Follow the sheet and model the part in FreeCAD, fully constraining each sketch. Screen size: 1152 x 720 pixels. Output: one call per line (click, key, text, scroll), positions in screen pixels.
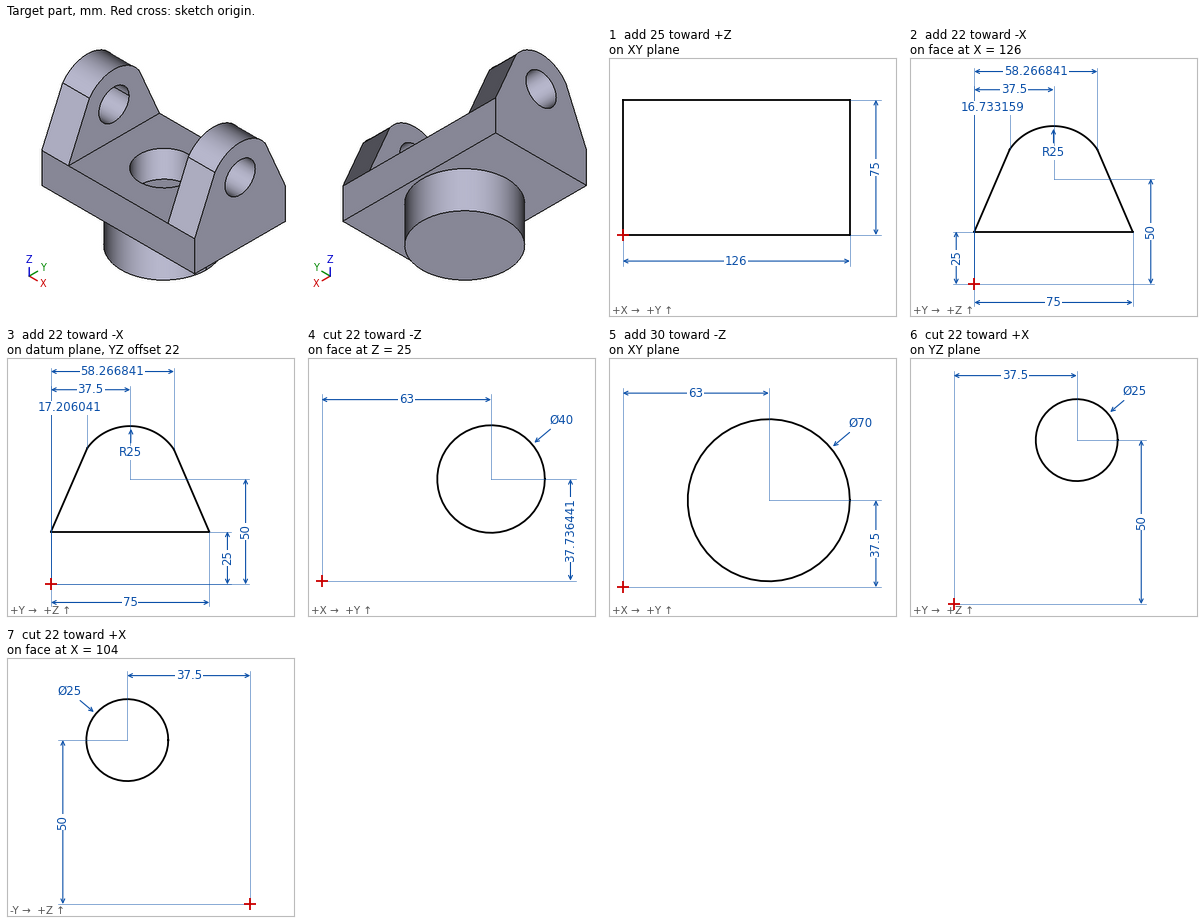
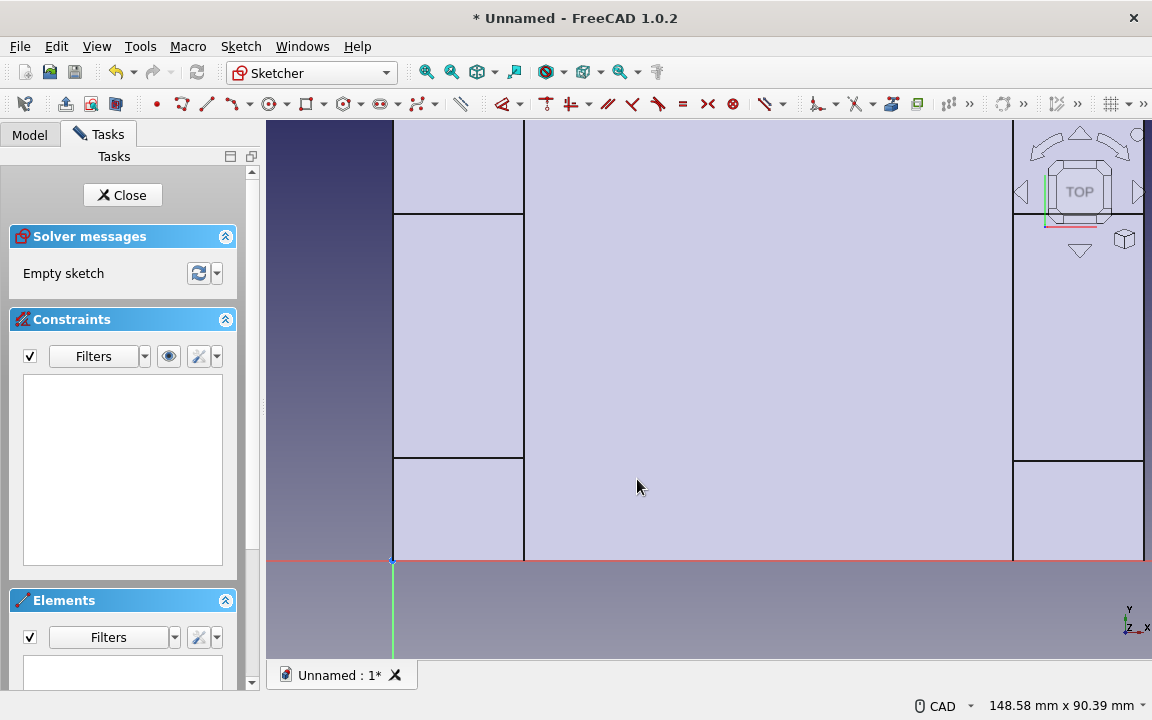
click(268, 104)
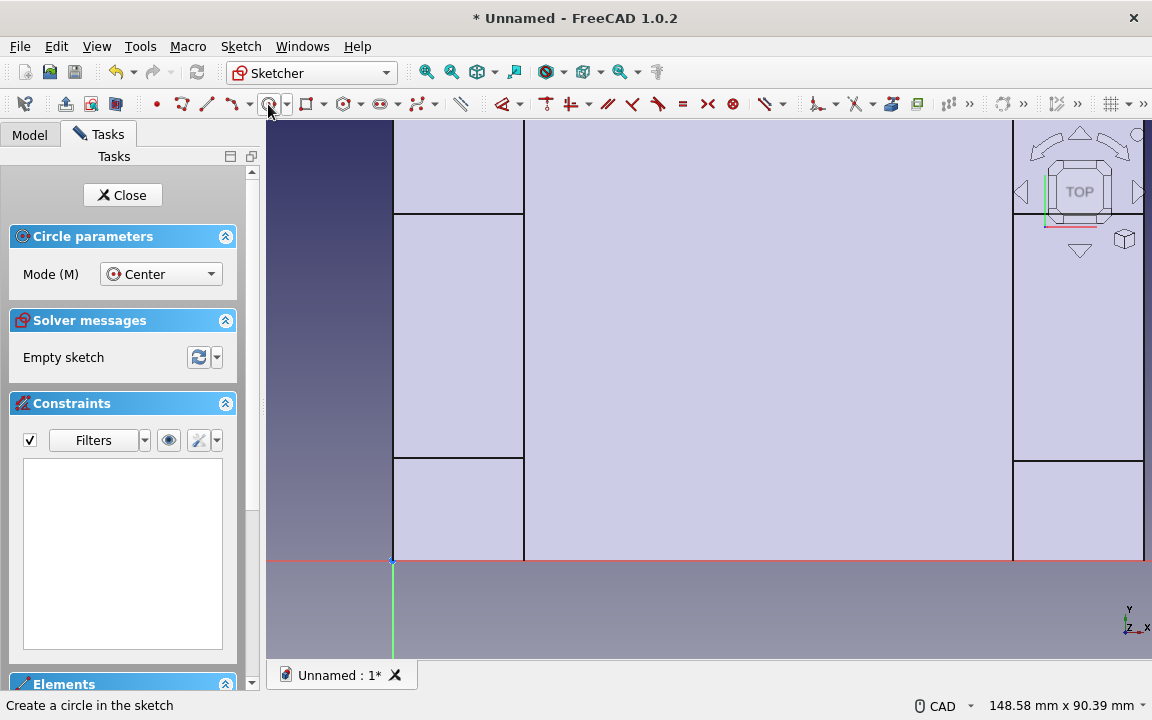
click(768, 336)
move(853, 252)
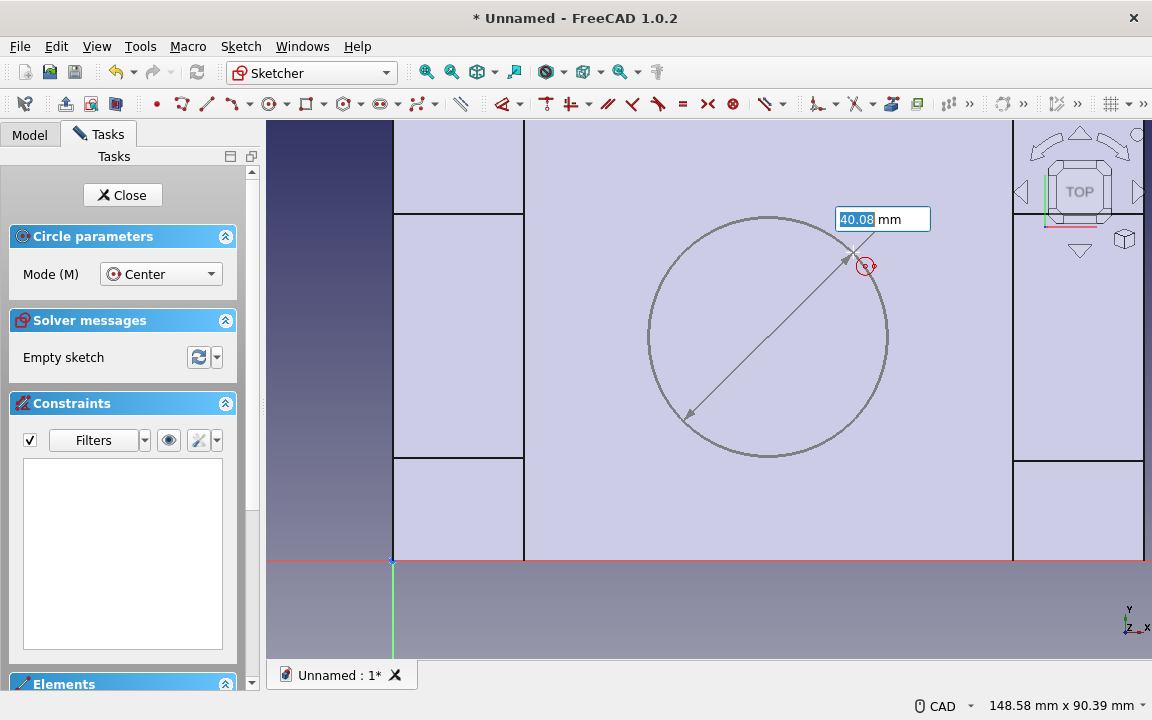
text(40)
key(Return)
key(Escape)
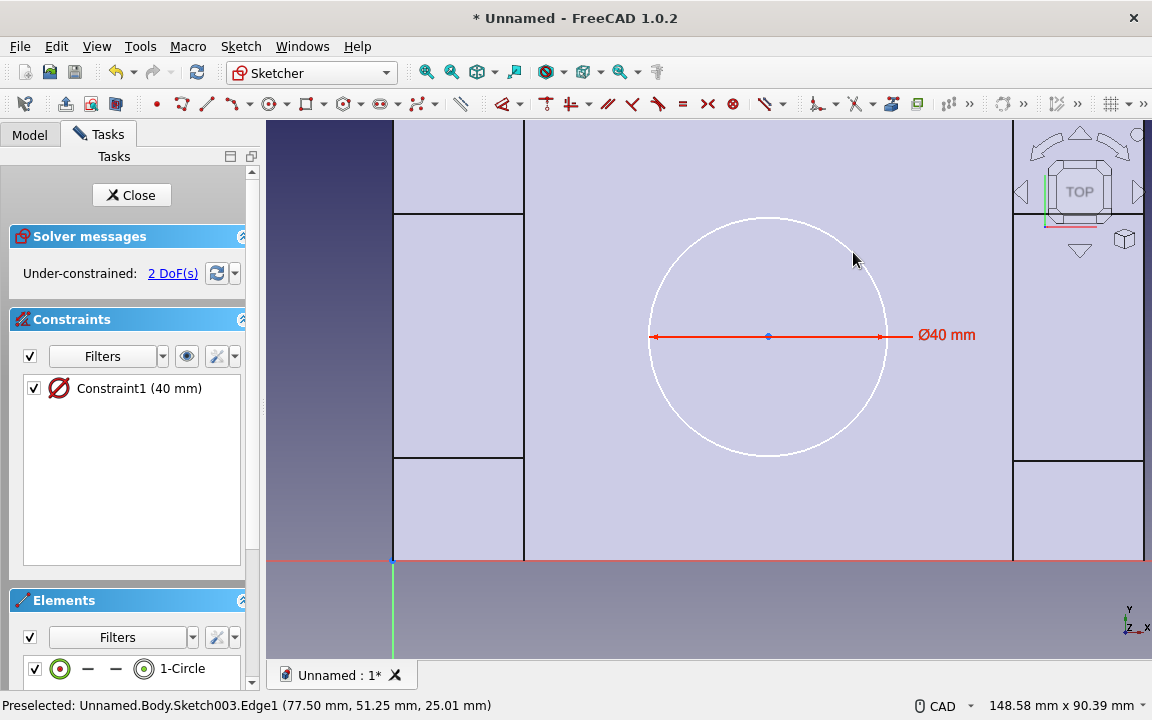
click(502, 104)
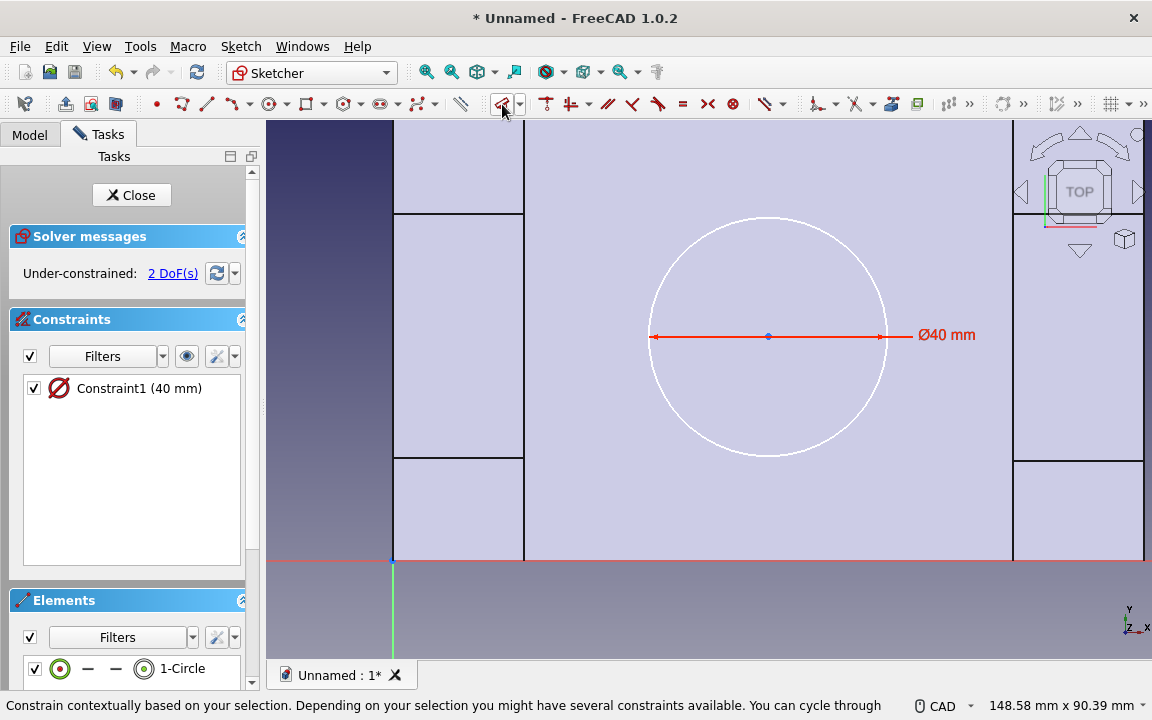
click(768, 337)
click(580, 595)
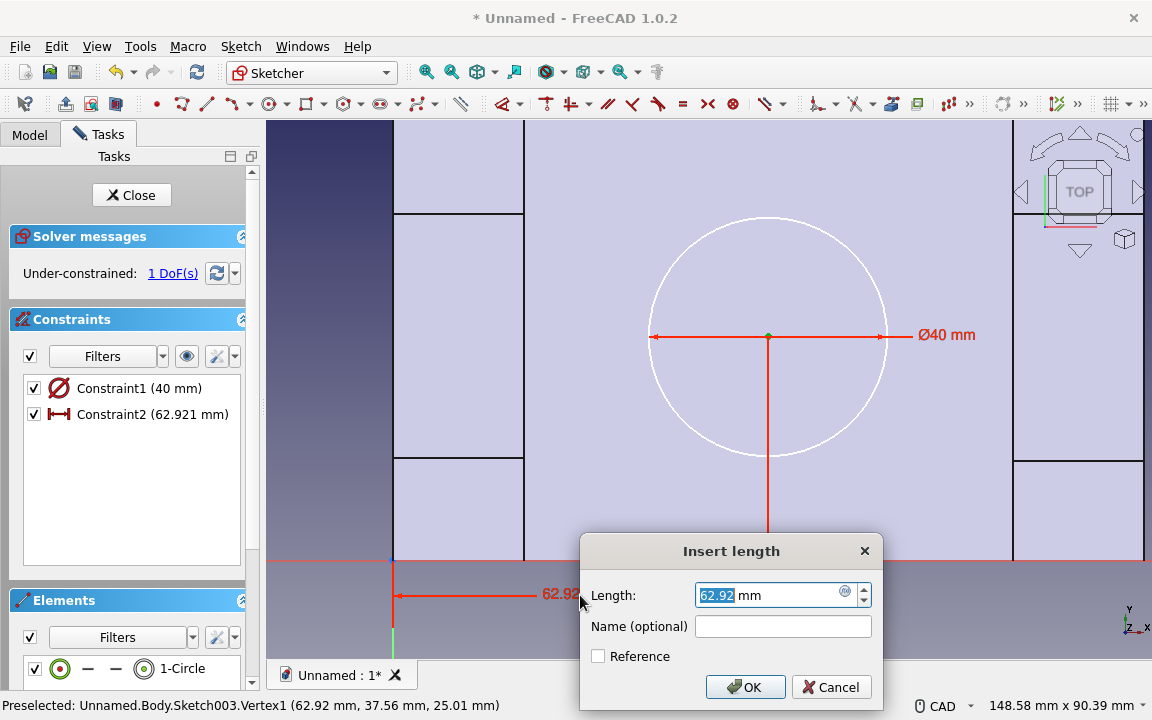
text(63)
key(Return)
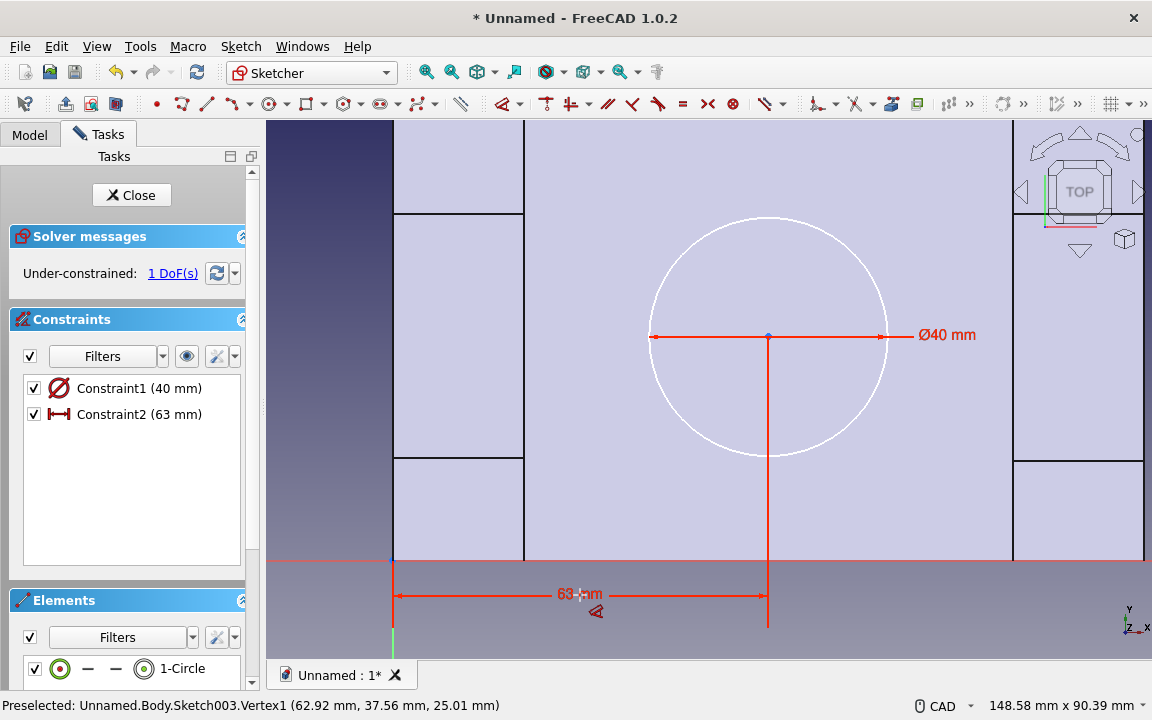
click(768, 337)
click(359, 449)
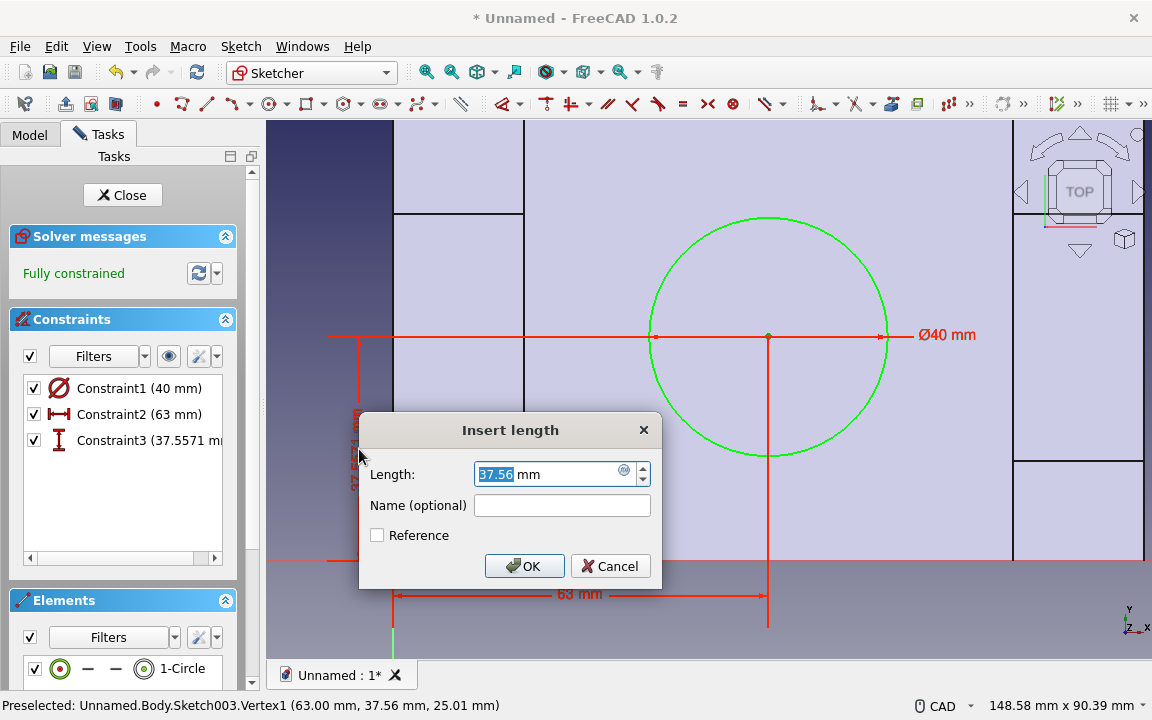
text(37.736441)
key(Return)
key(Escape)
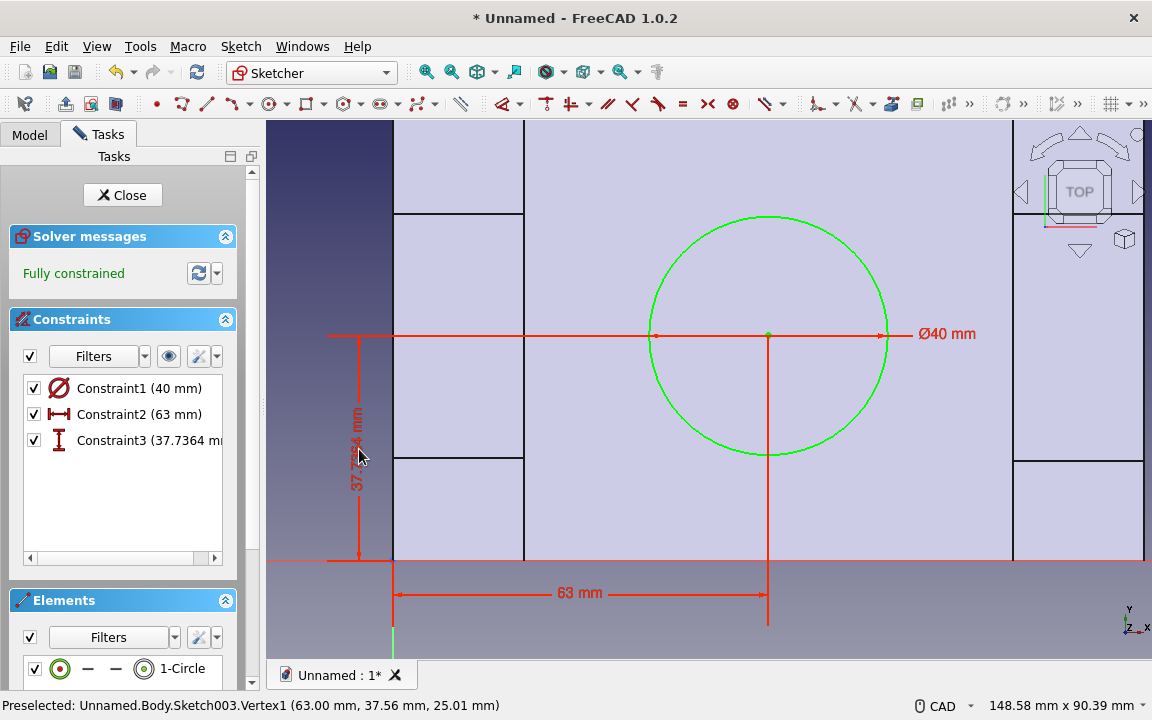
click(123, 195)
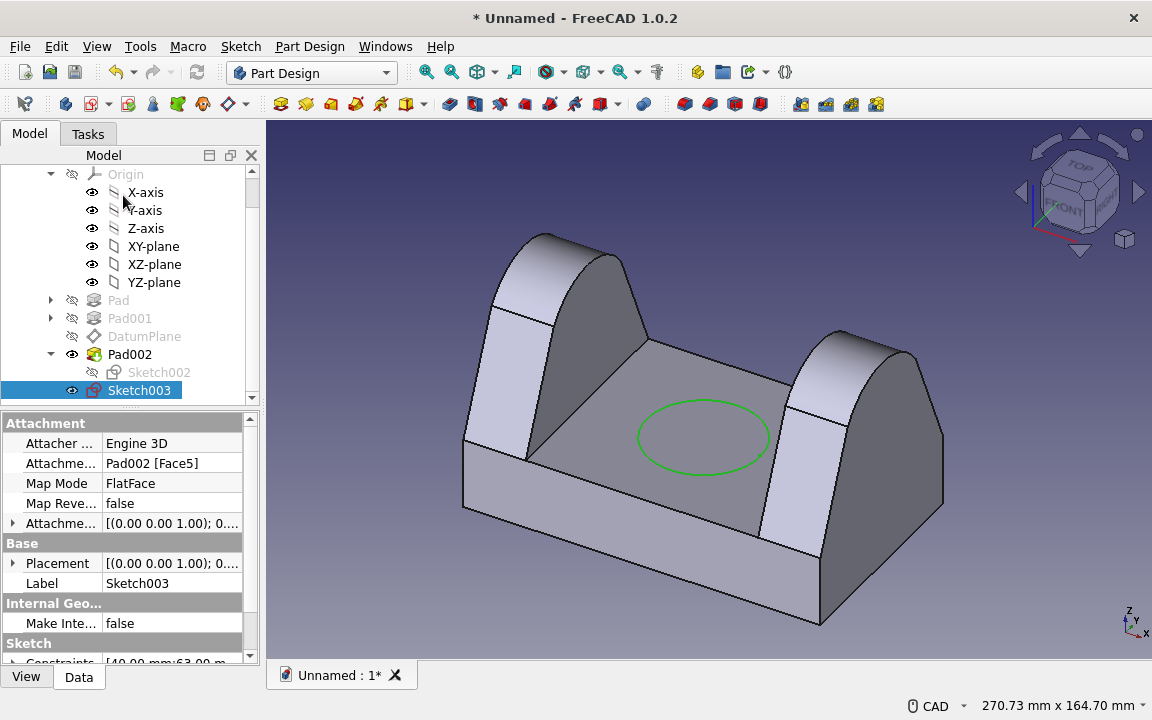
click(450, 104)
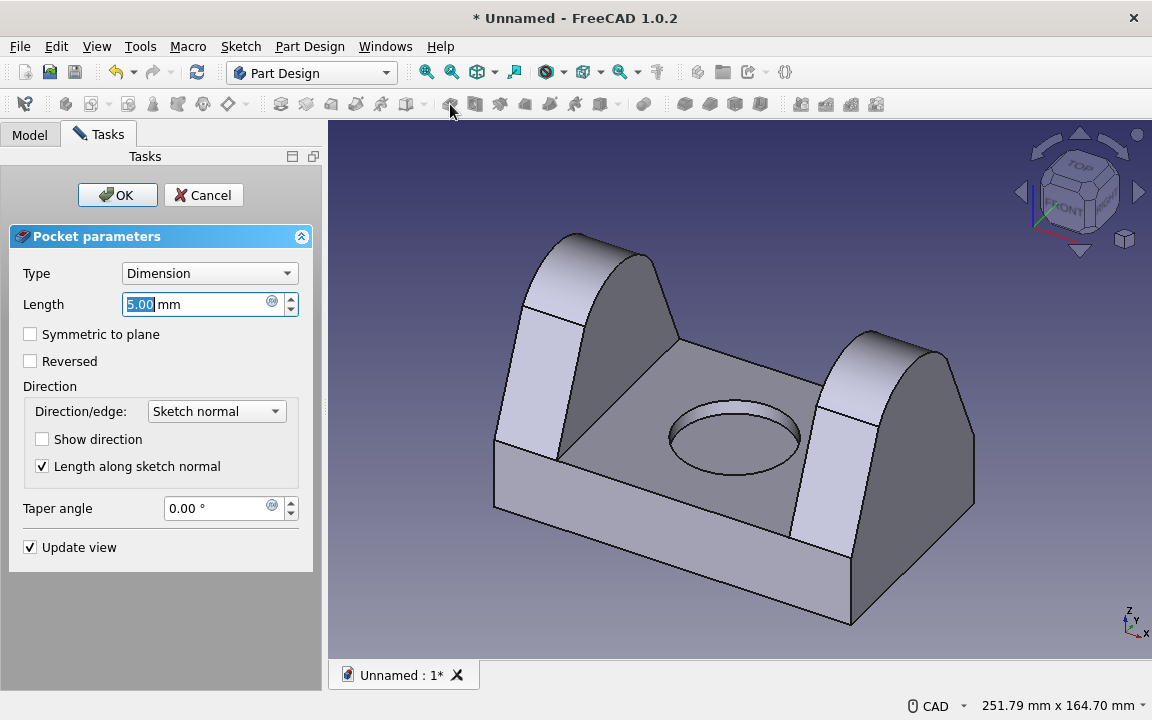
text(22)
key(Tab)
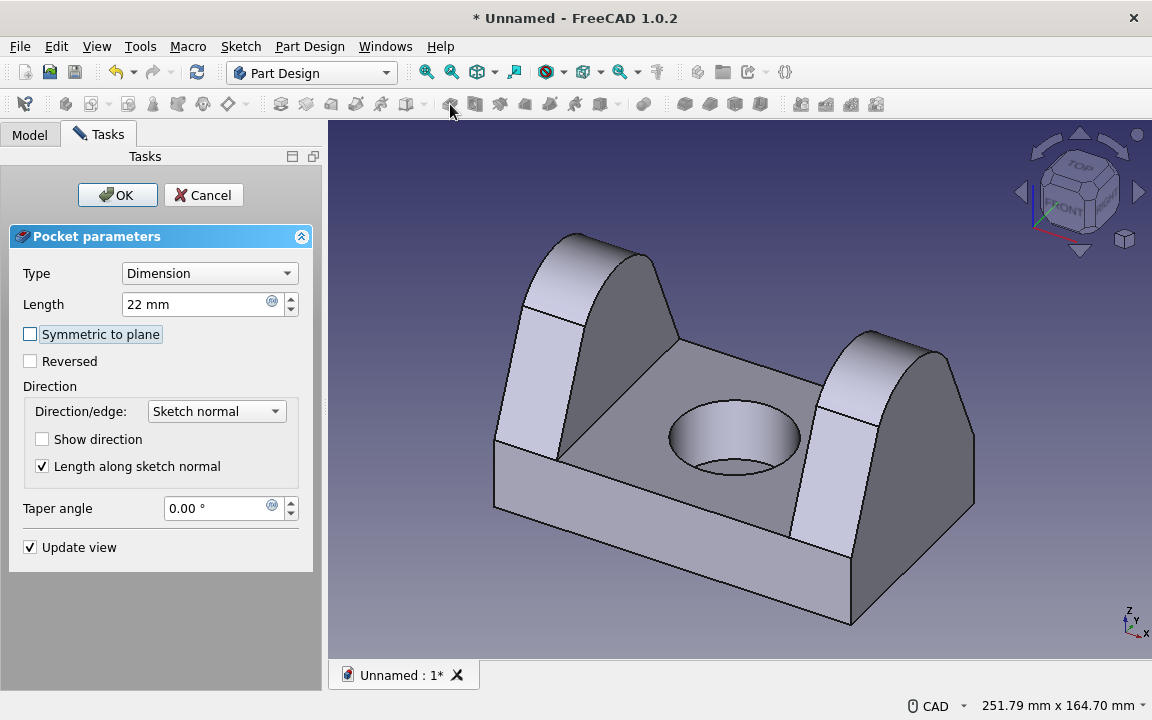
click(118, 195)